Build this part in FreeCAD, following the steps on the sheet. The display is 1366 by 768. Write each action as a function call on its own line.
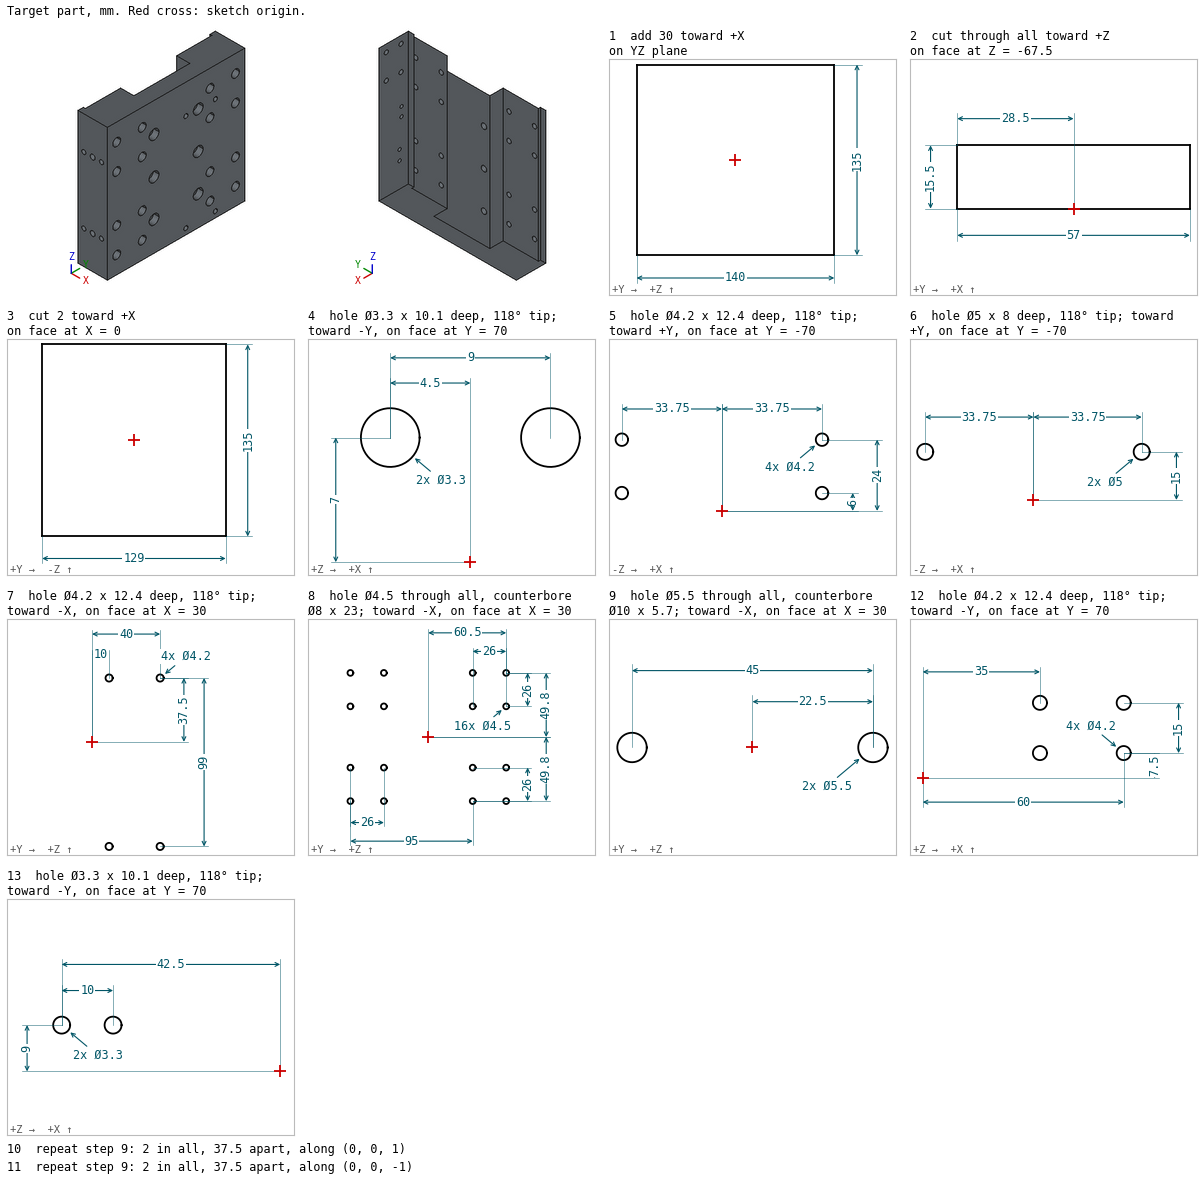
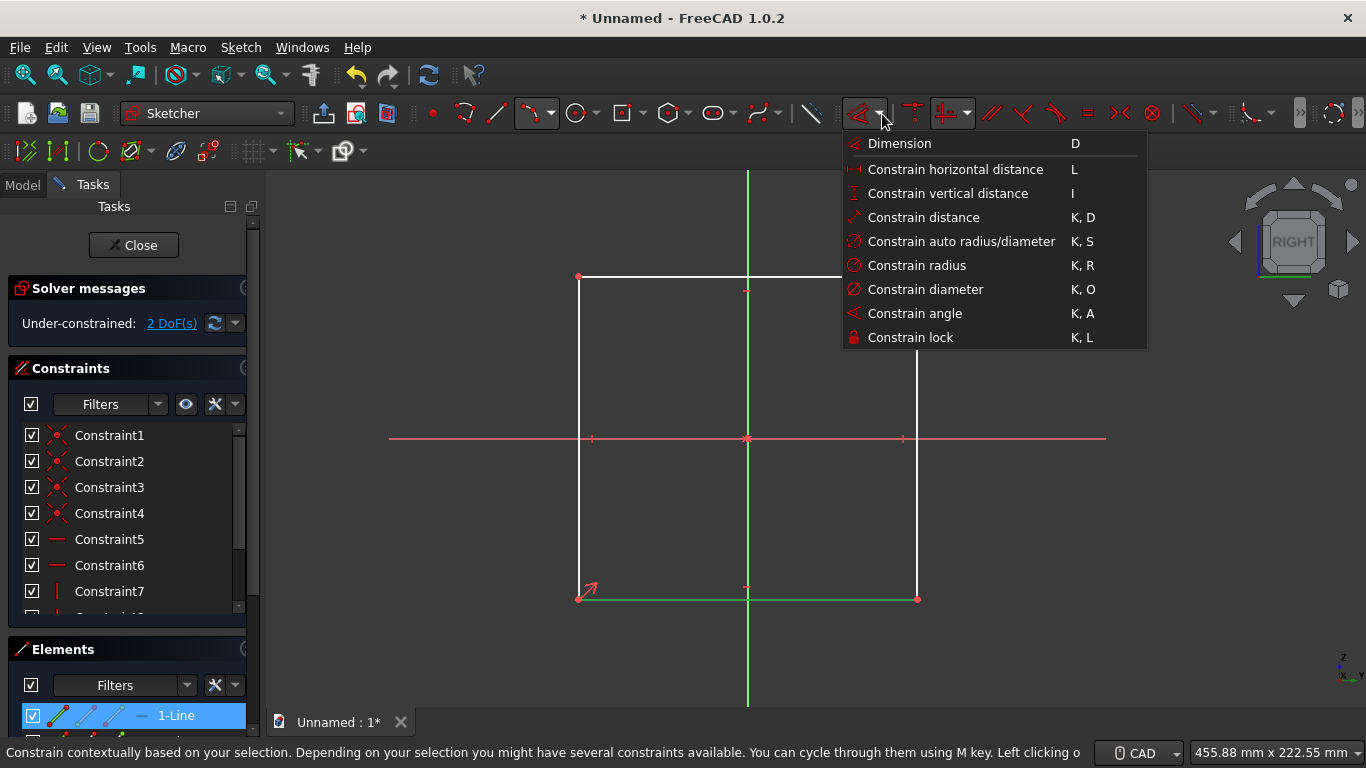
click(995, 169)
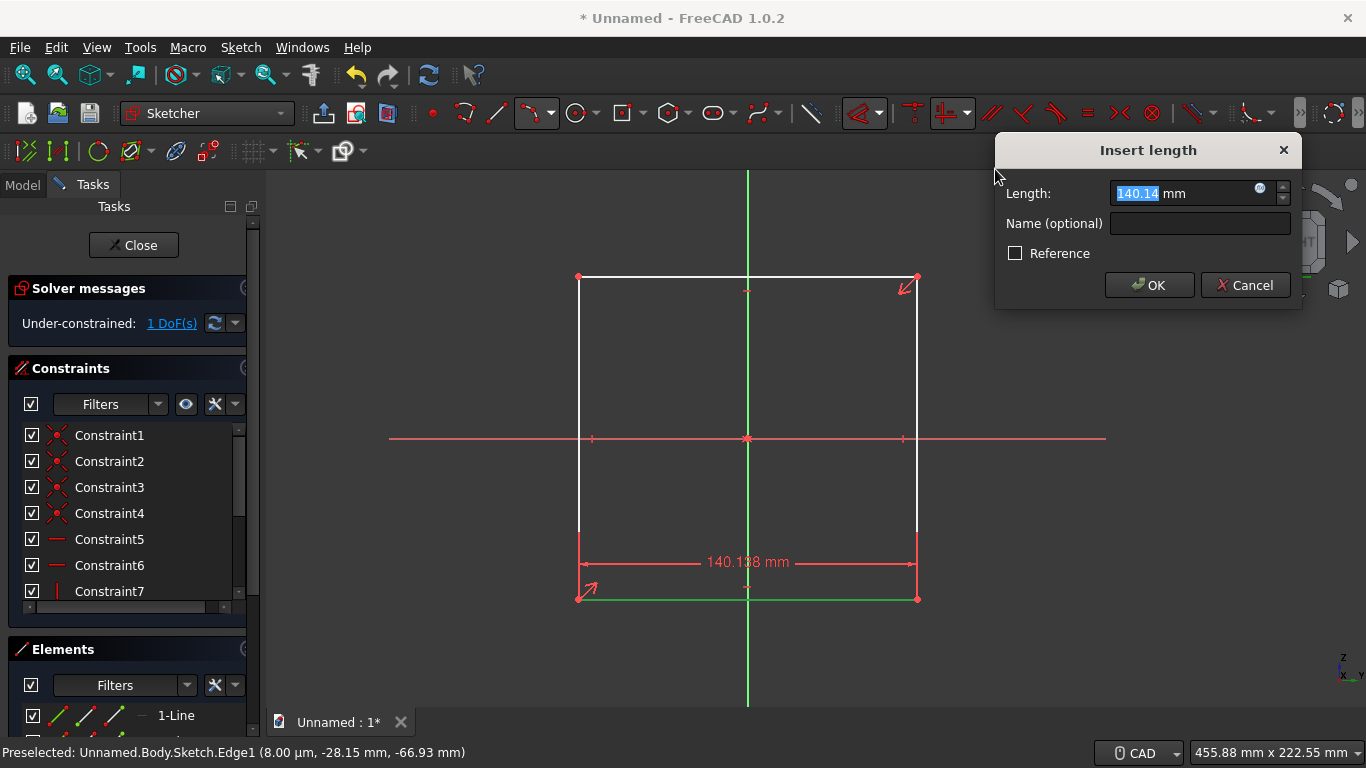
text(140)
key(Return)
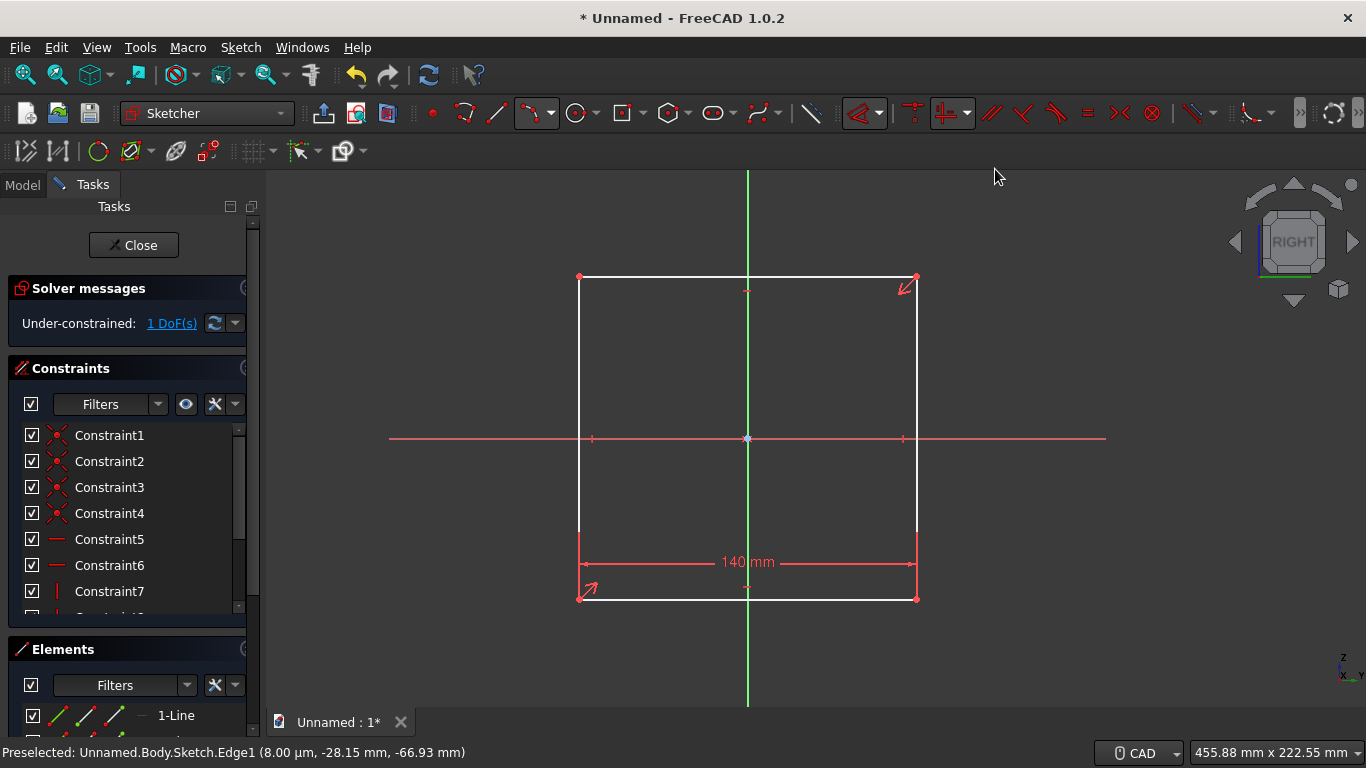
click(917, 503)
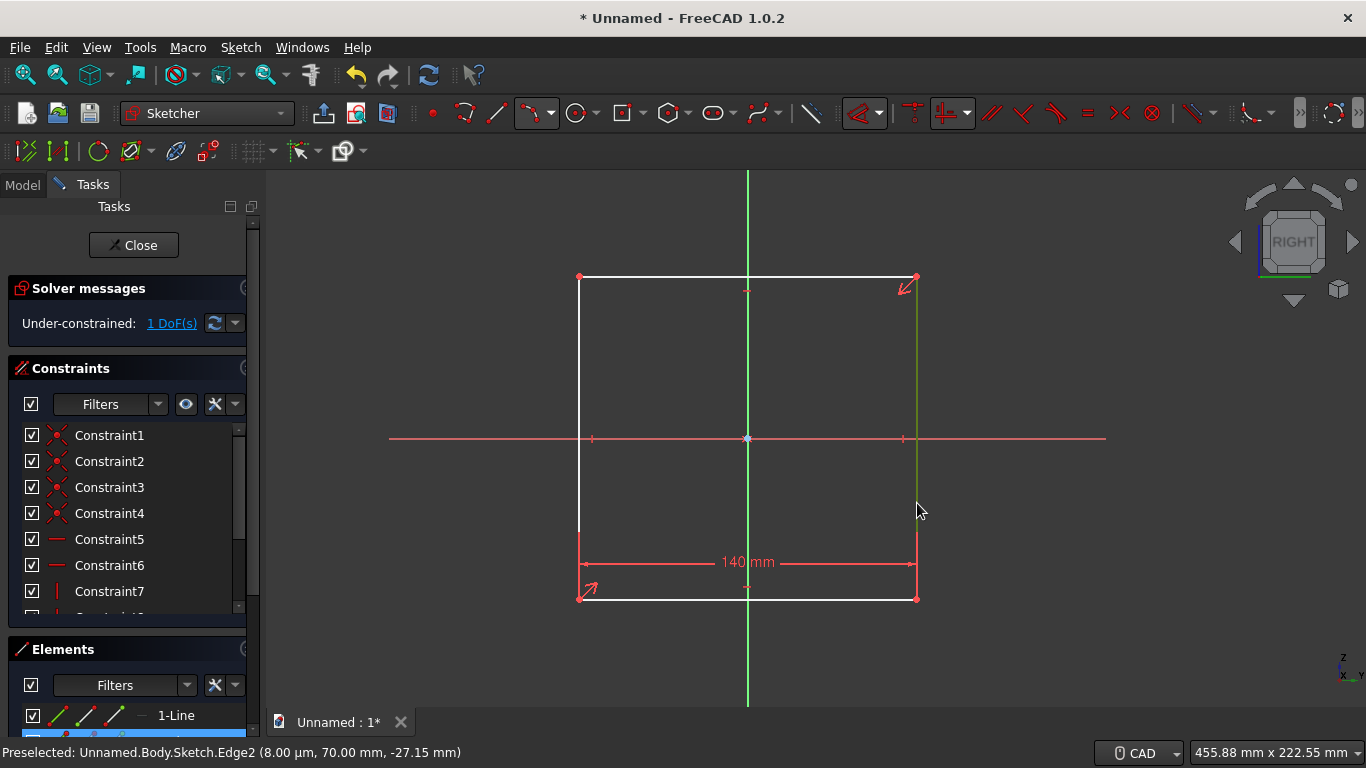
click(882, 114)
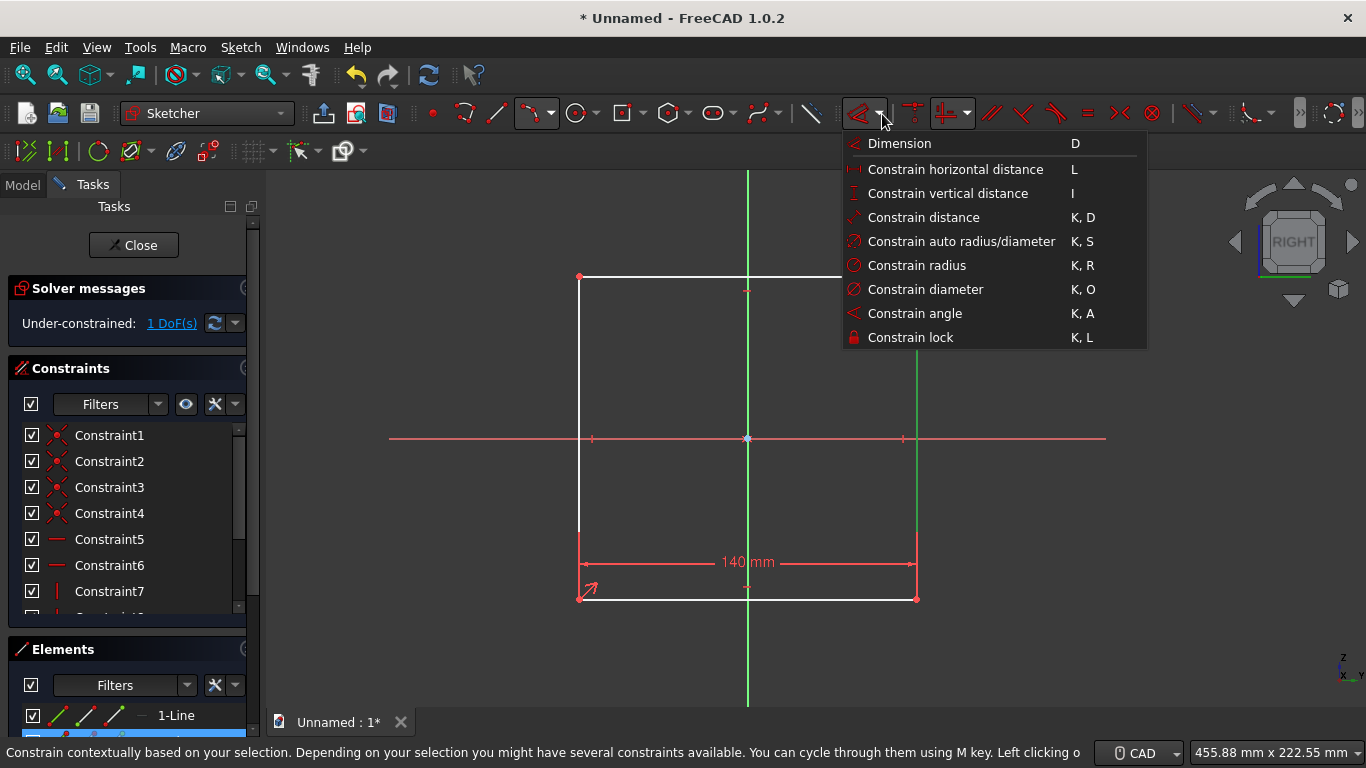
click(995, 193)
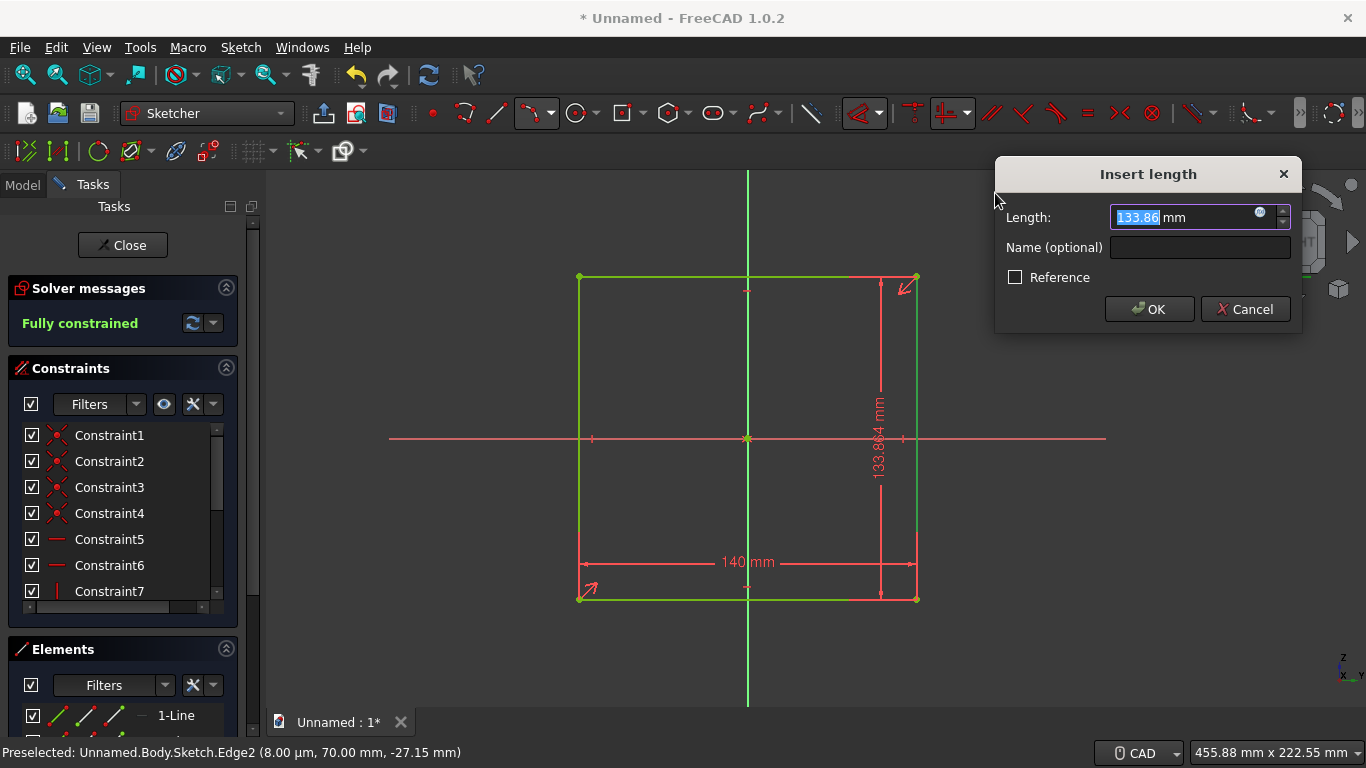
text(135)
key(Return)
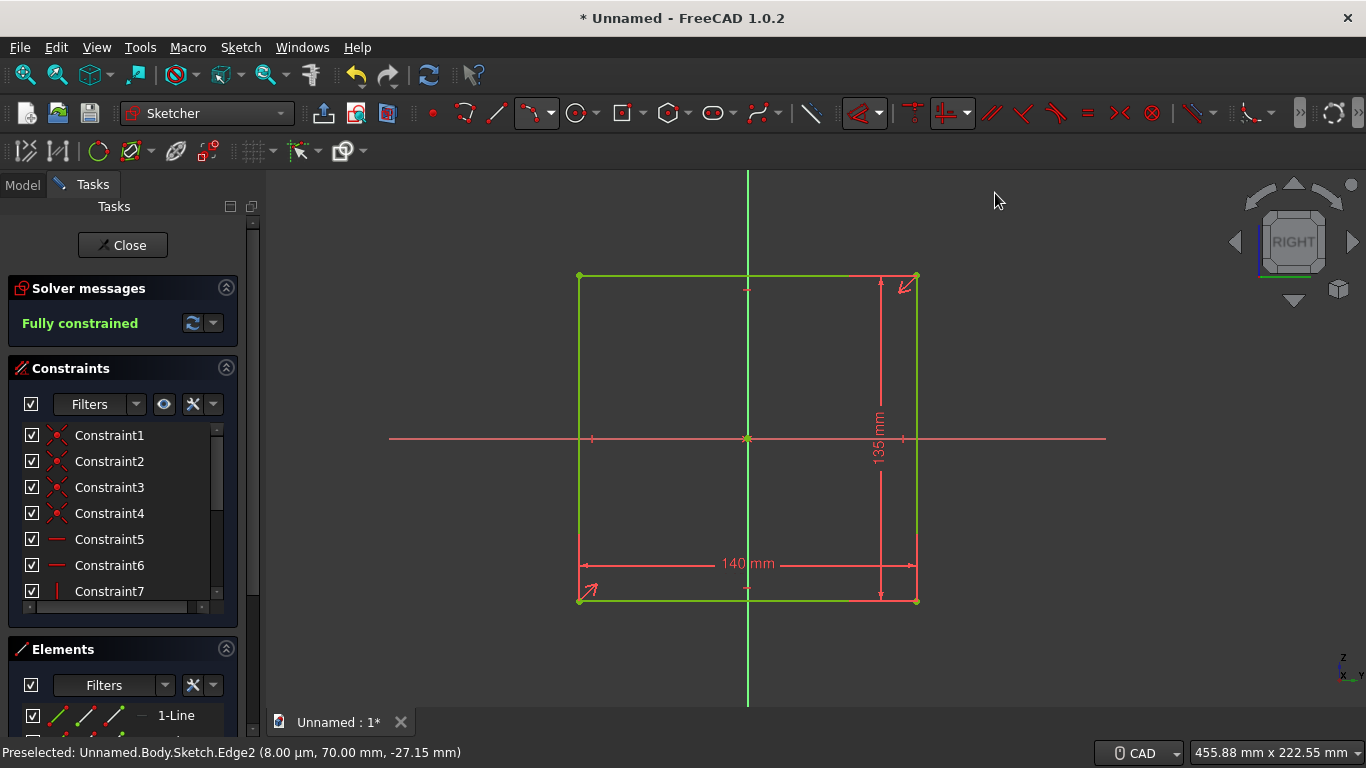
click(123, 245)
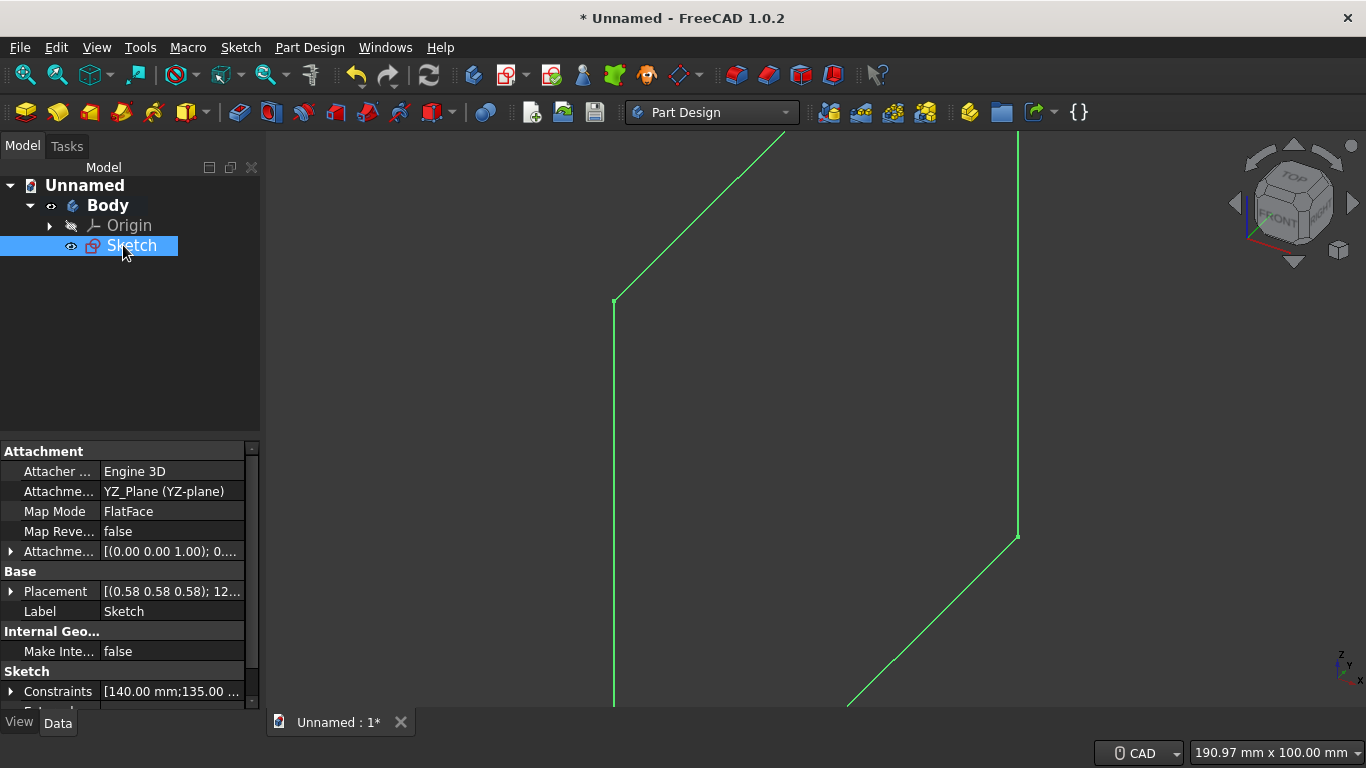
click(26, 112)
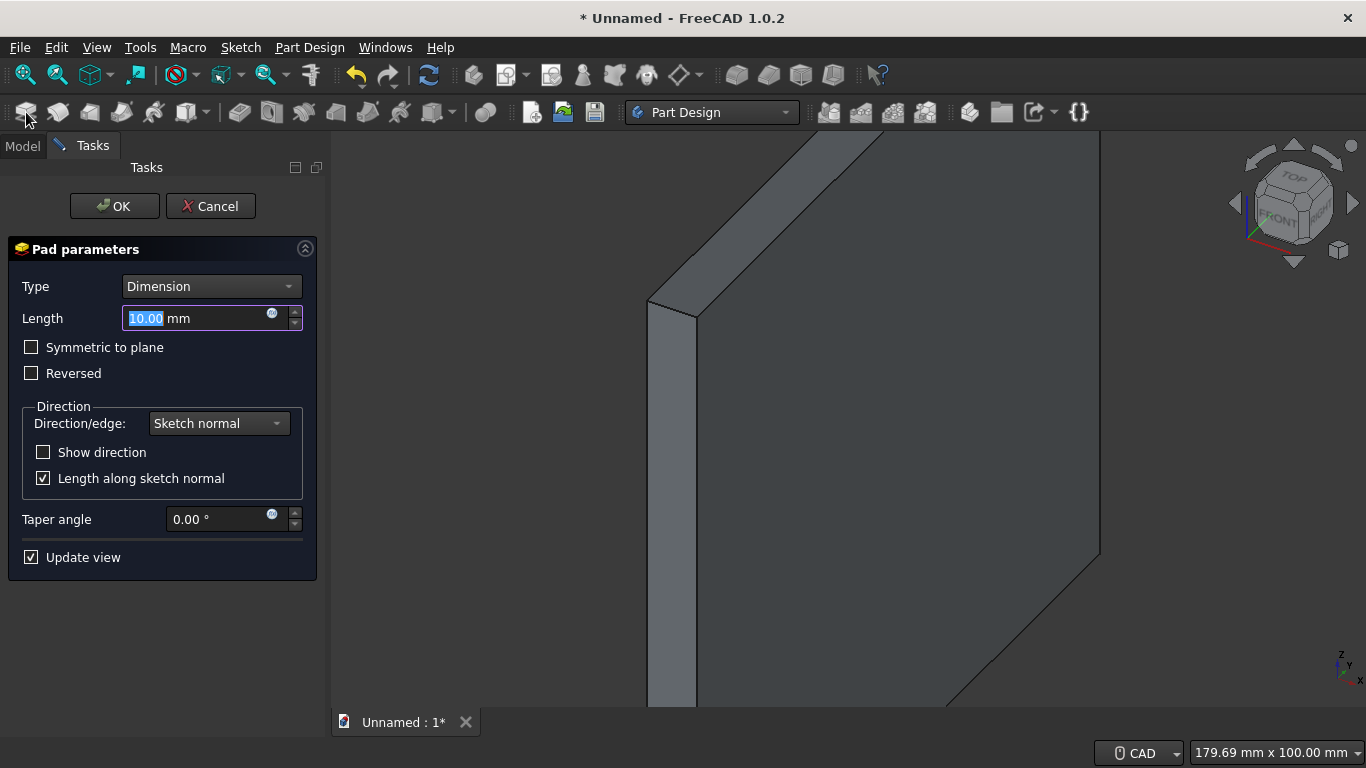
text(30)
key(Tab)